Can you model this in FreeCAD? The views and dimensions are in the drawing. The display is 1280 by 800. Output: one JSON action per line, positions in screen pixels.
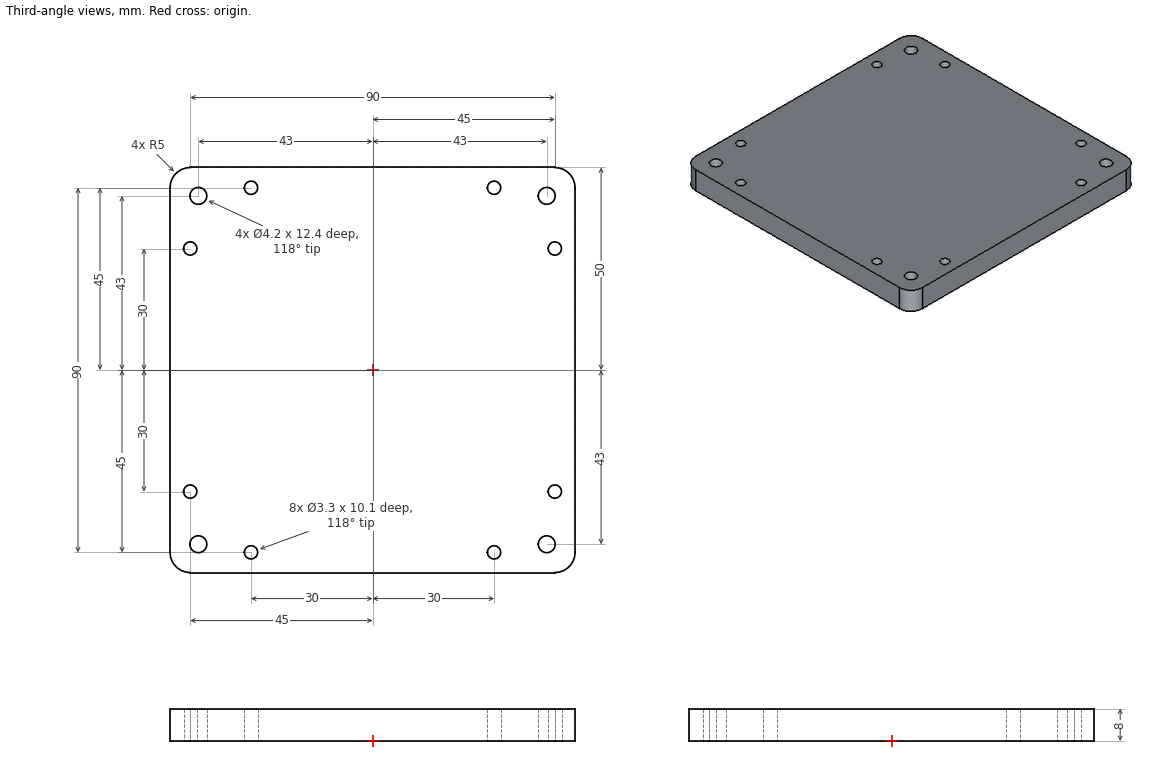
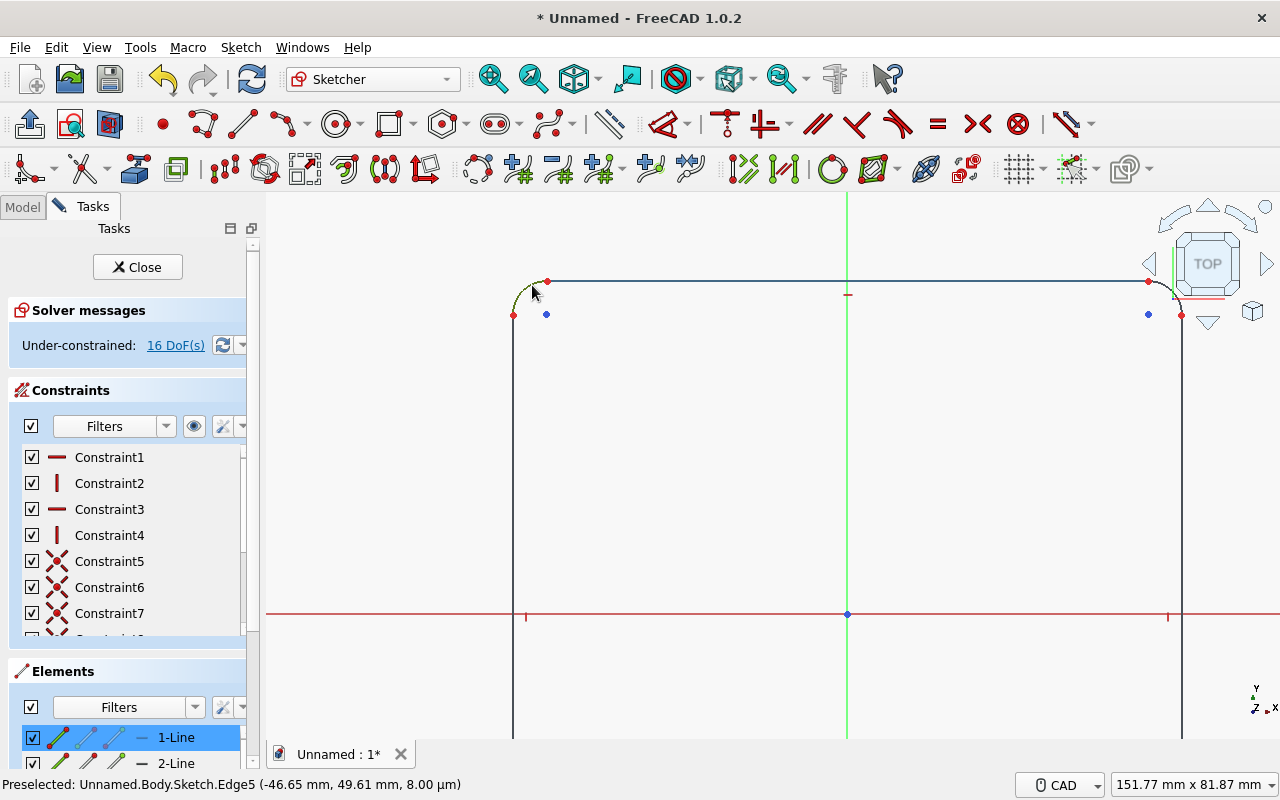
{"action": "key", "text": "t"}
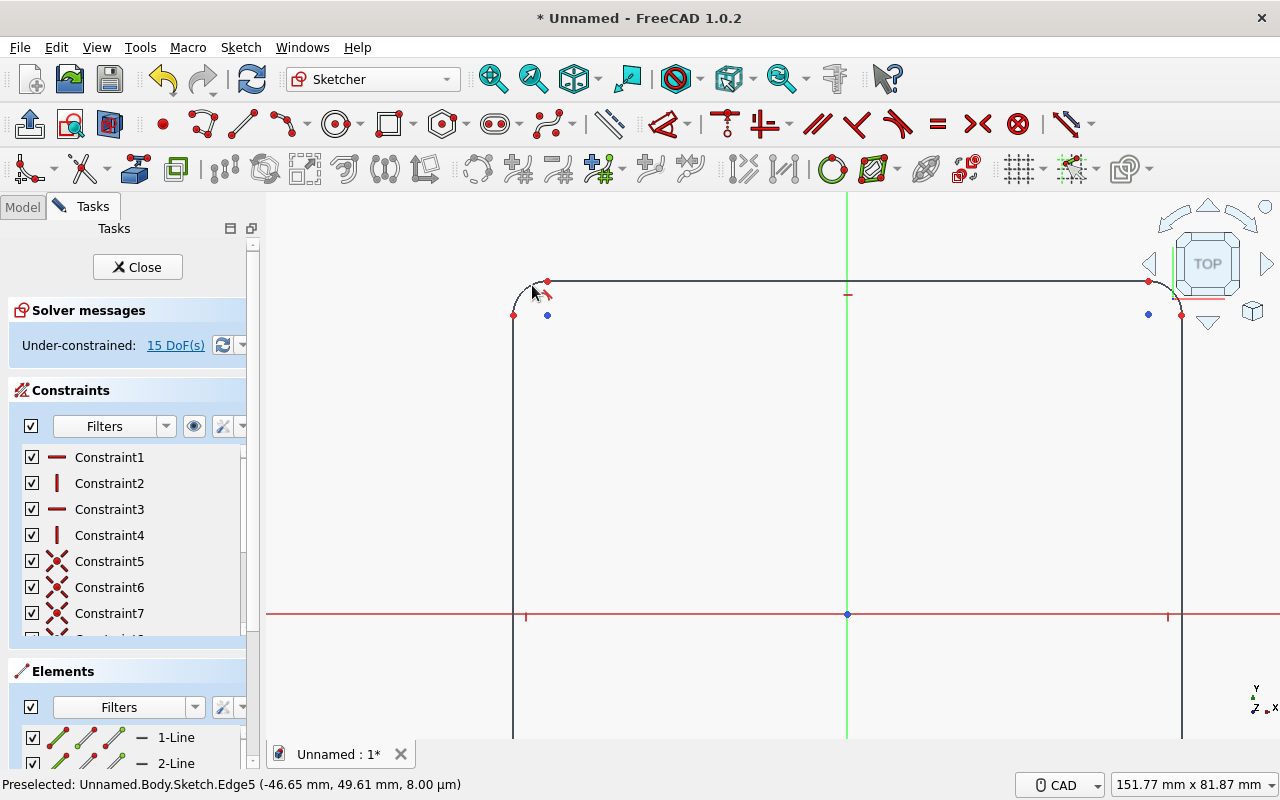
{"action": "left_click", "coordinate": [969, 281]}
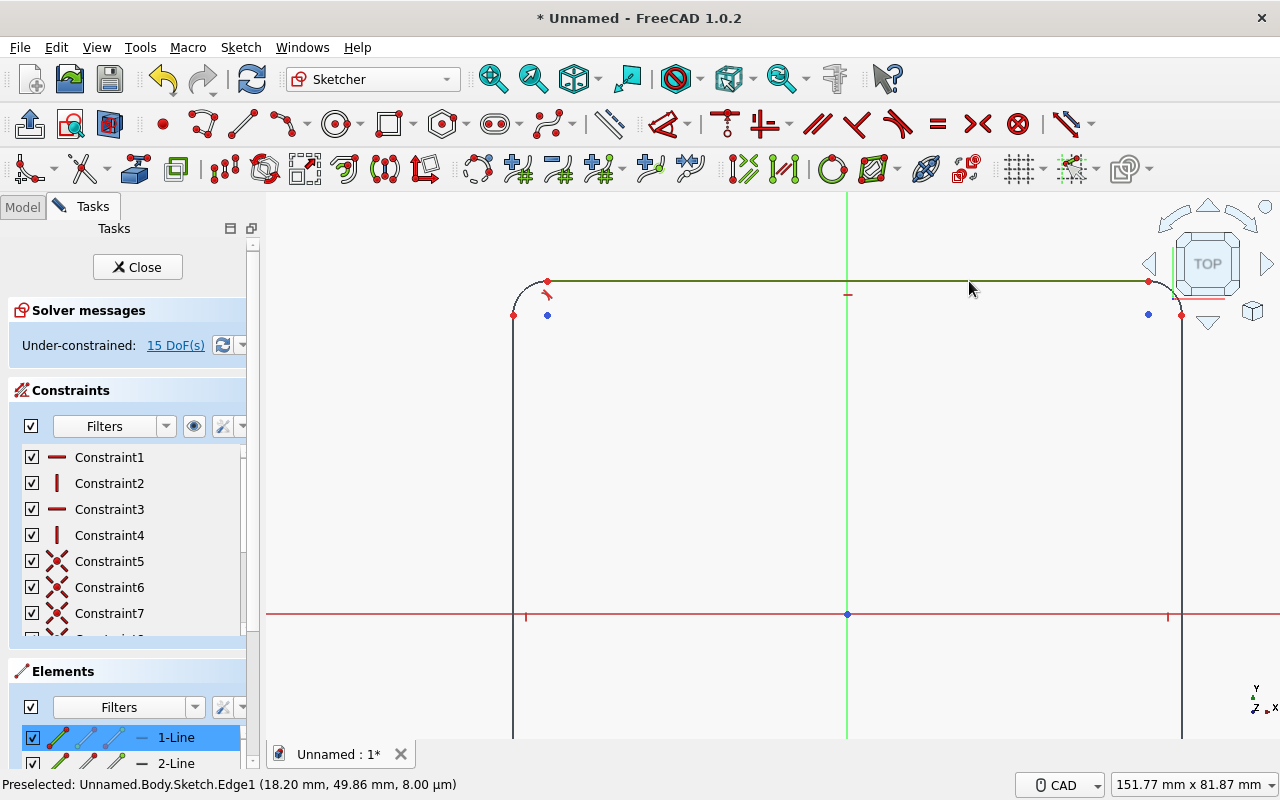
{"action": "scroll", "coordinate": [531, 284], "scroll_direction": "down", "scroll_amount": 3}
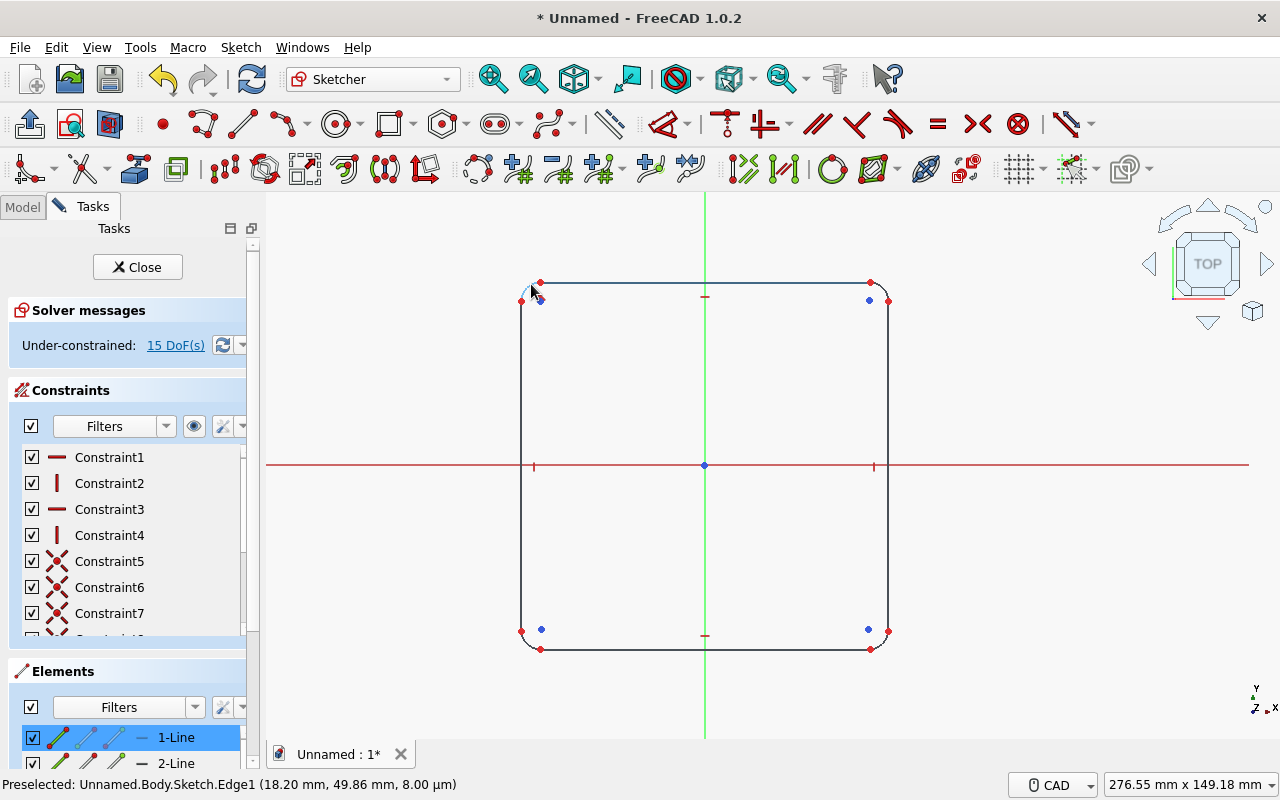
{"action": "scroll", "coordinate": [887, 293], "scroll_direction": "up", "scroll_amount": 3}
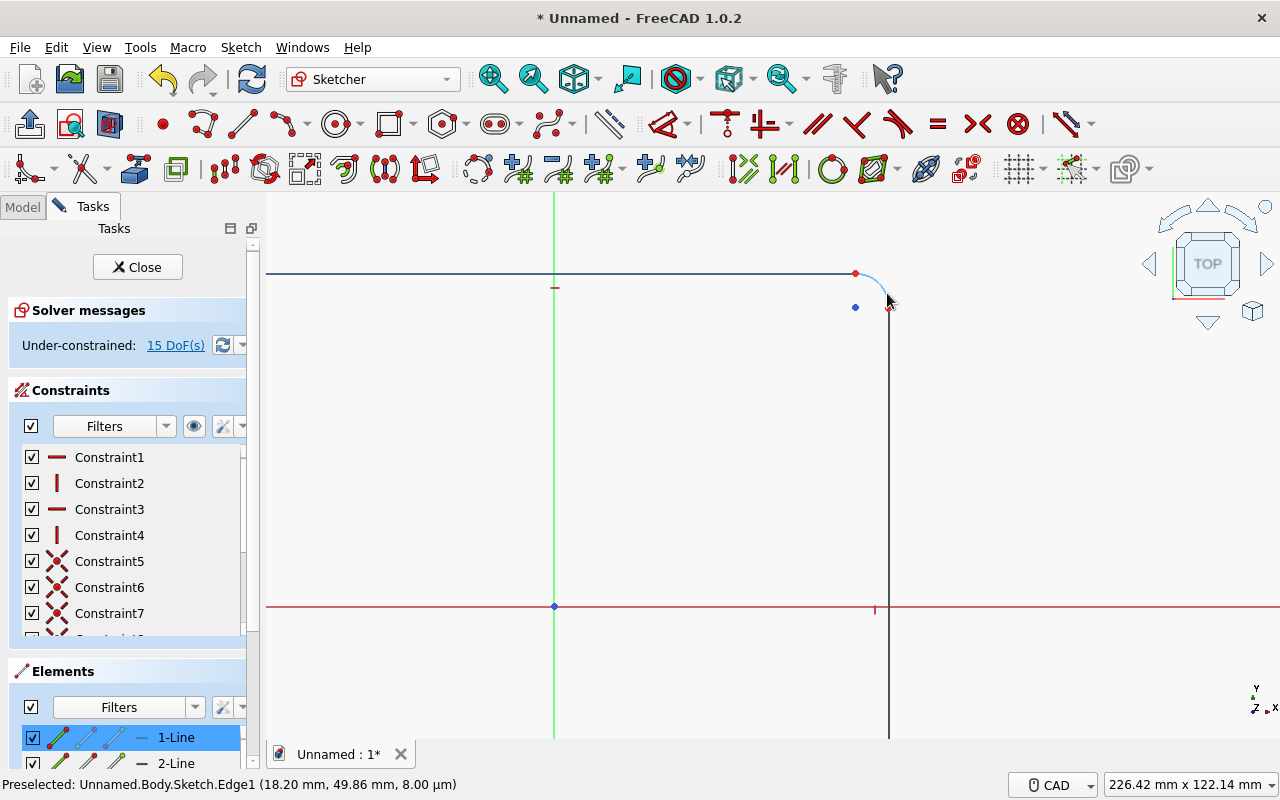
{"action": "left_click", "coordinate": [886, 293]}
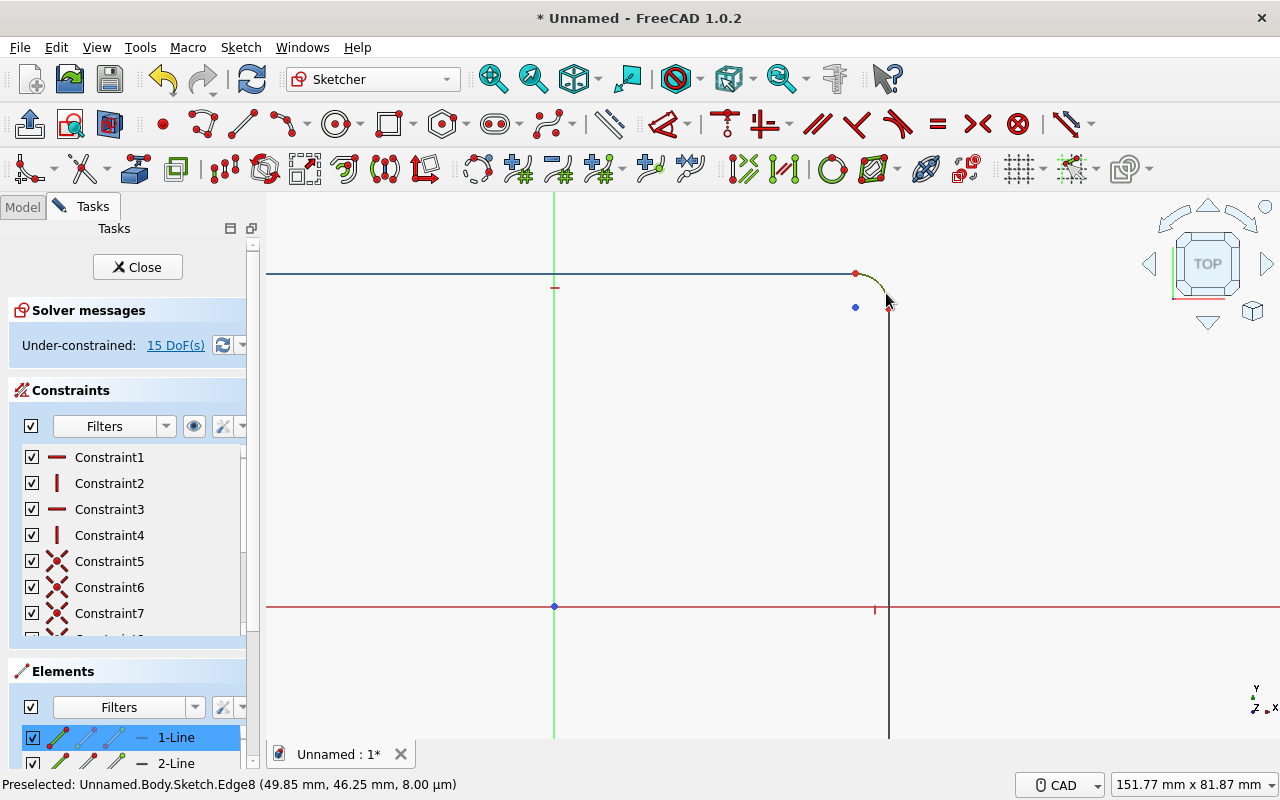
{"action": "key", "text": "t"}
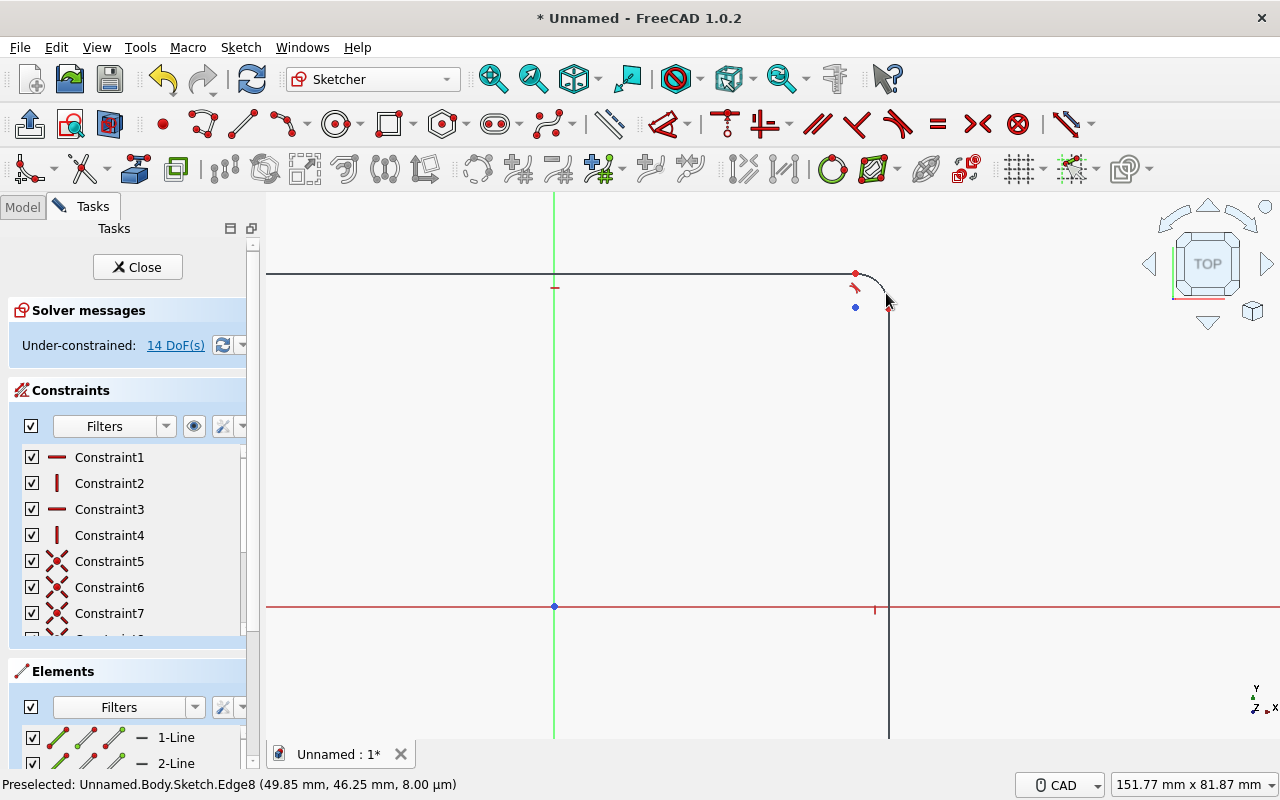
{"action": "scroll", "coordinate": [887, 293], "scroll_direction": "down", "scroll_amount": 3}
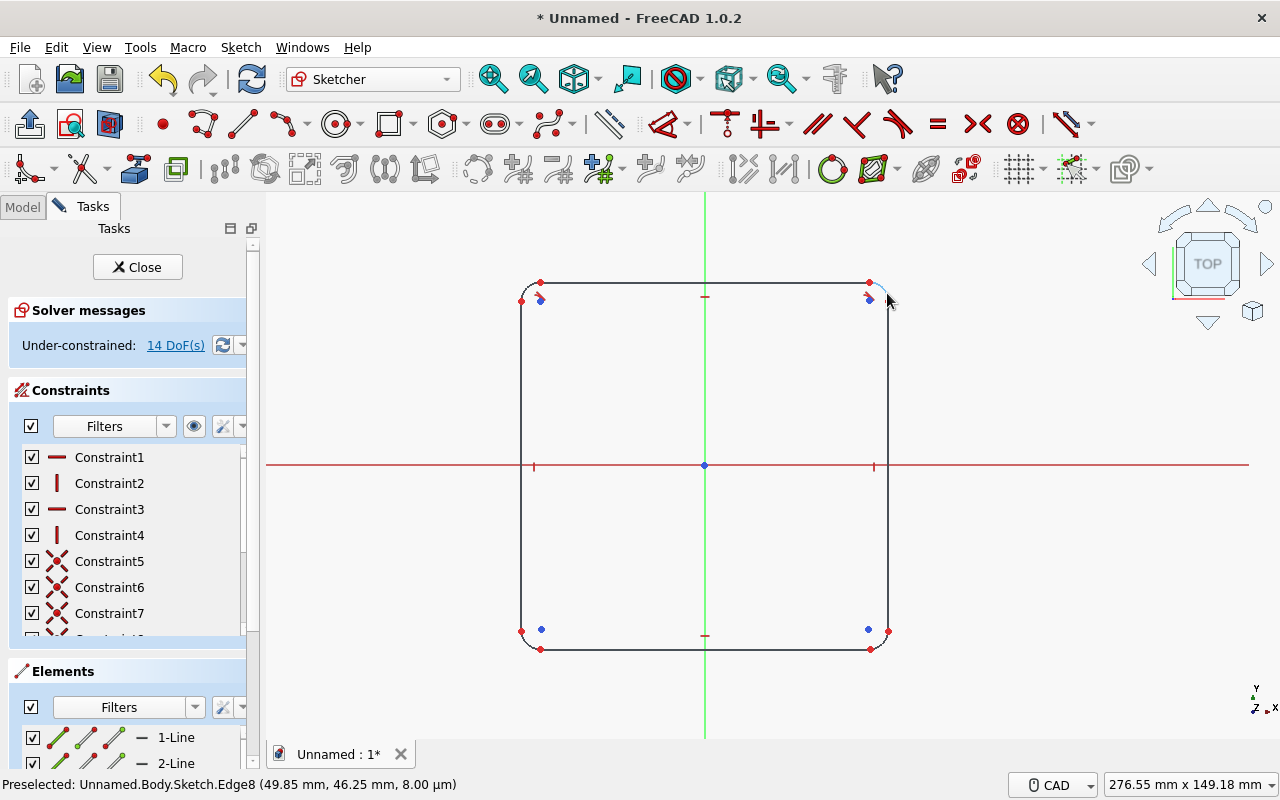
{"action": "left_click", "coordinate": [521, 401]}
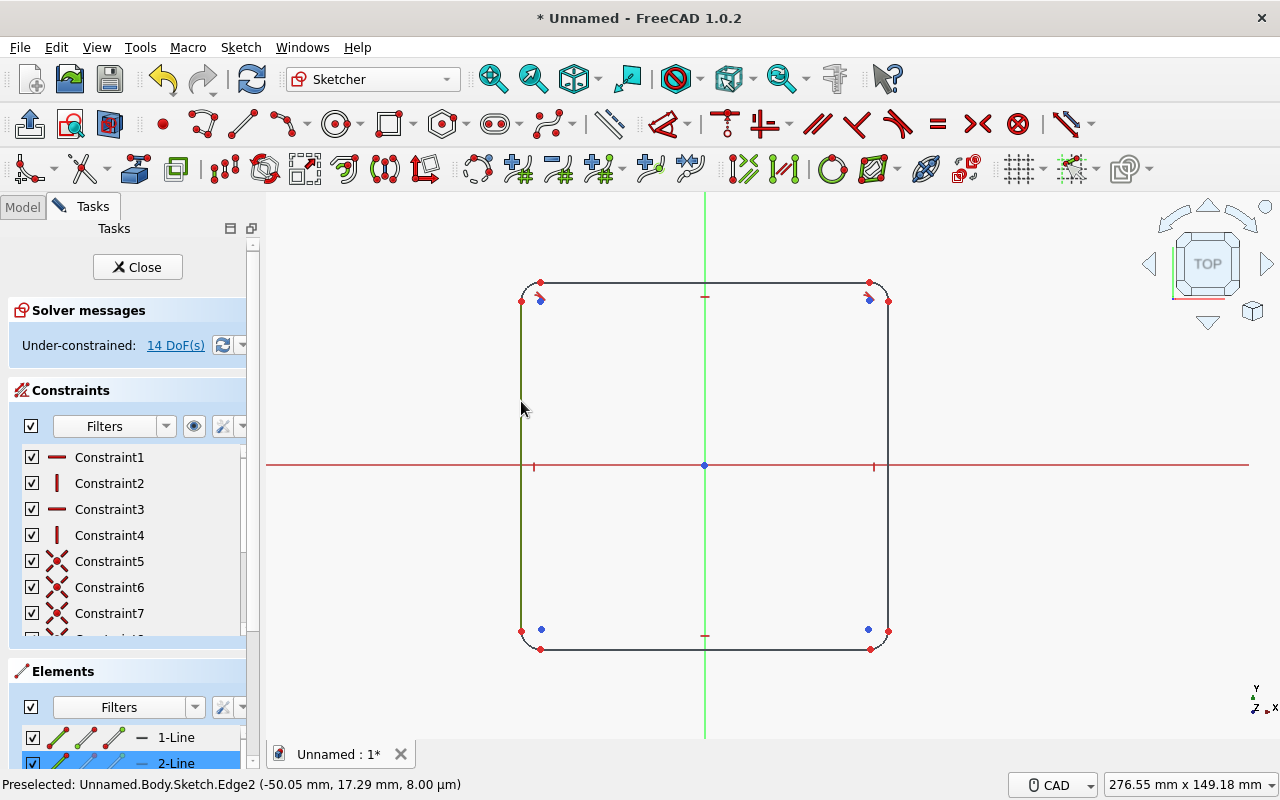
{"action": "left_click", "coordinate": [527, 288]}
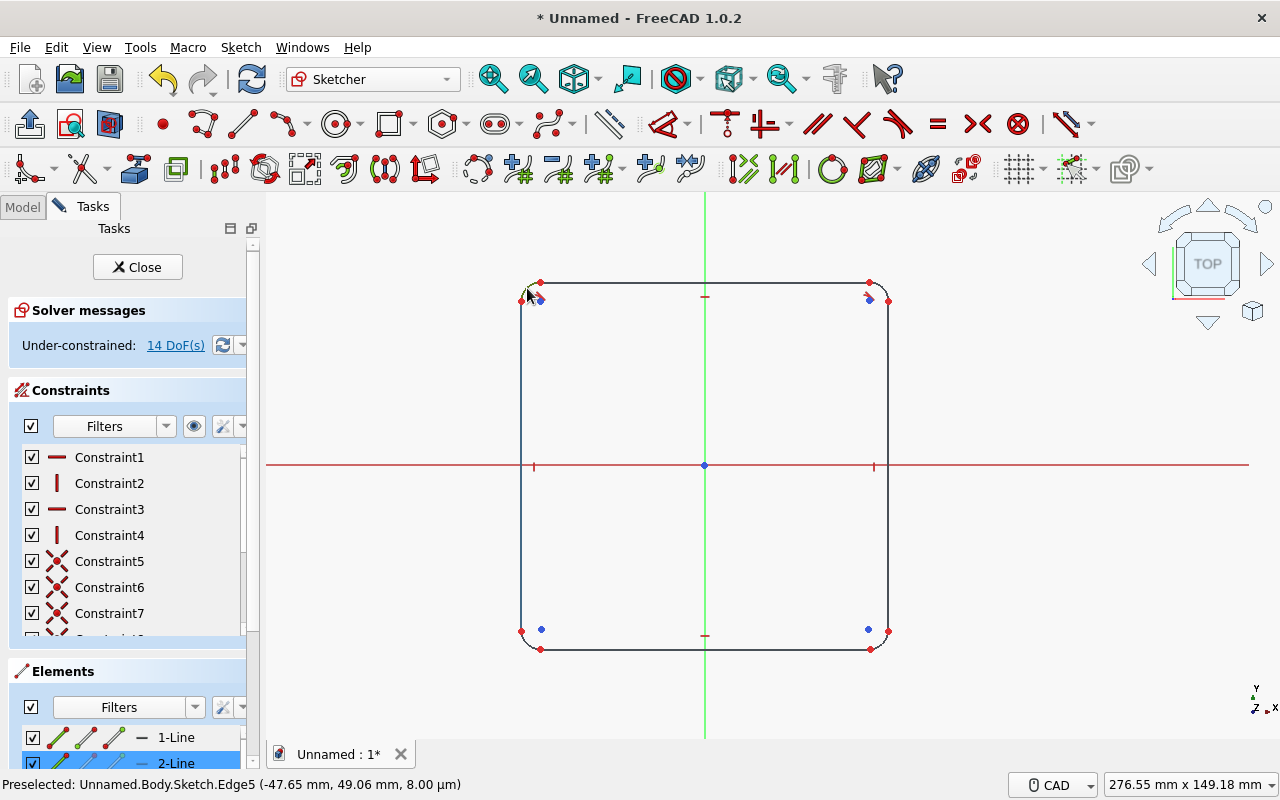
{"action": "left_click", "coordinate": [898, 124]}